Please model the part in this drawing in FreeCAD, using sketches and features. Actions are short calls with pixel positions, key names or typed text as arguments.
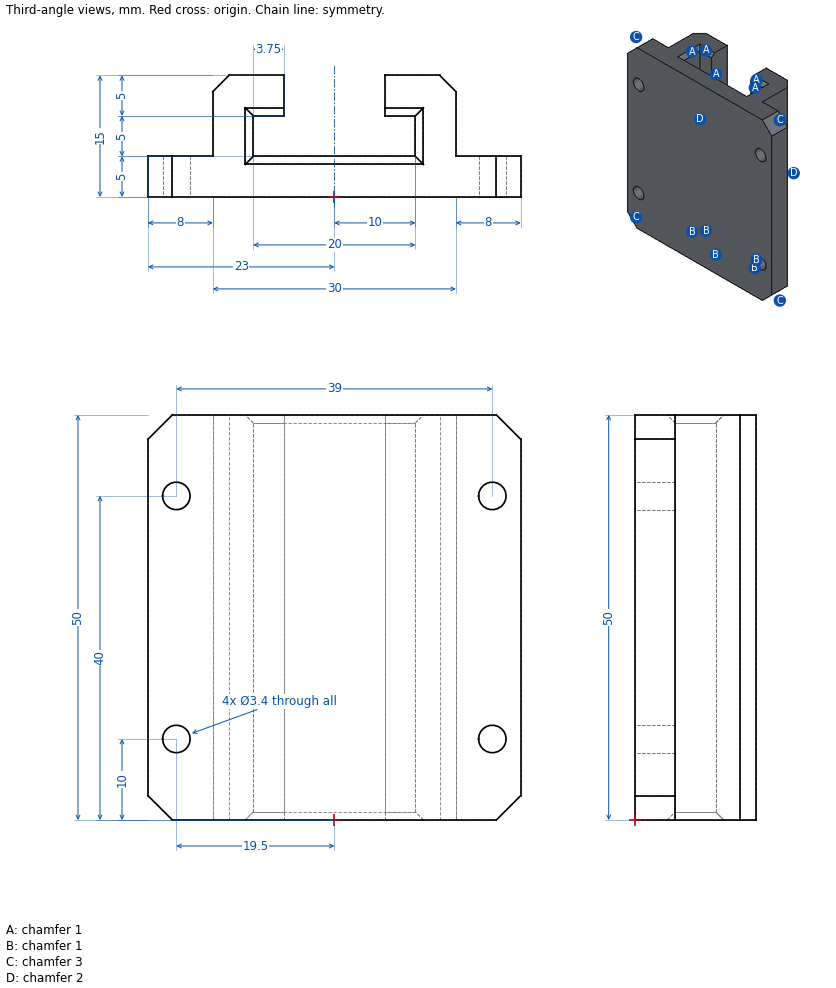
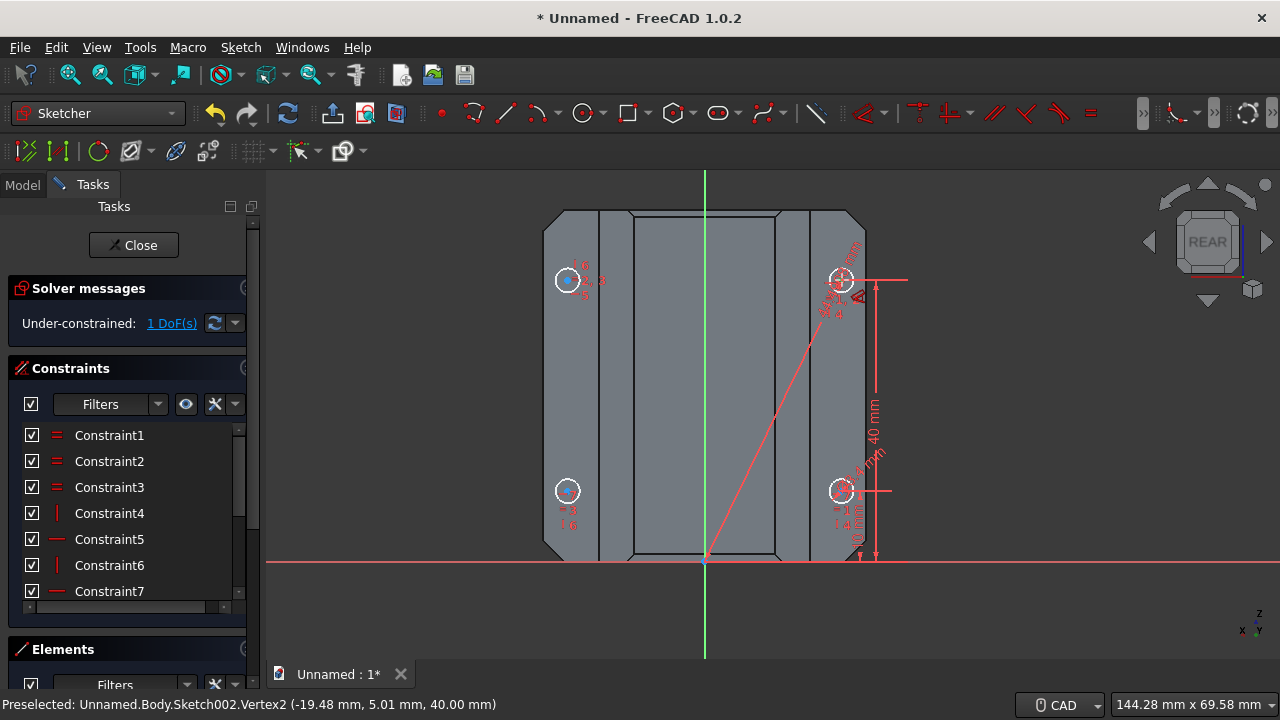
click(568, 280)
click(642, 246)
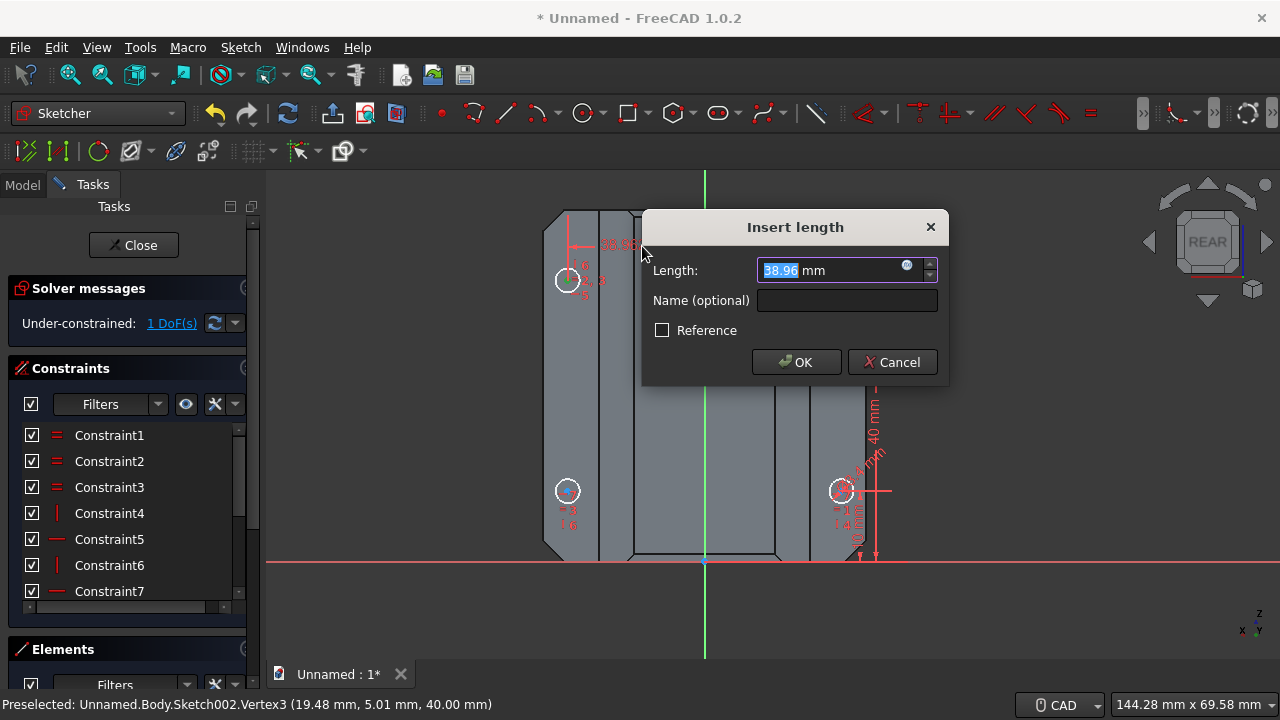
text(39)
key(Return)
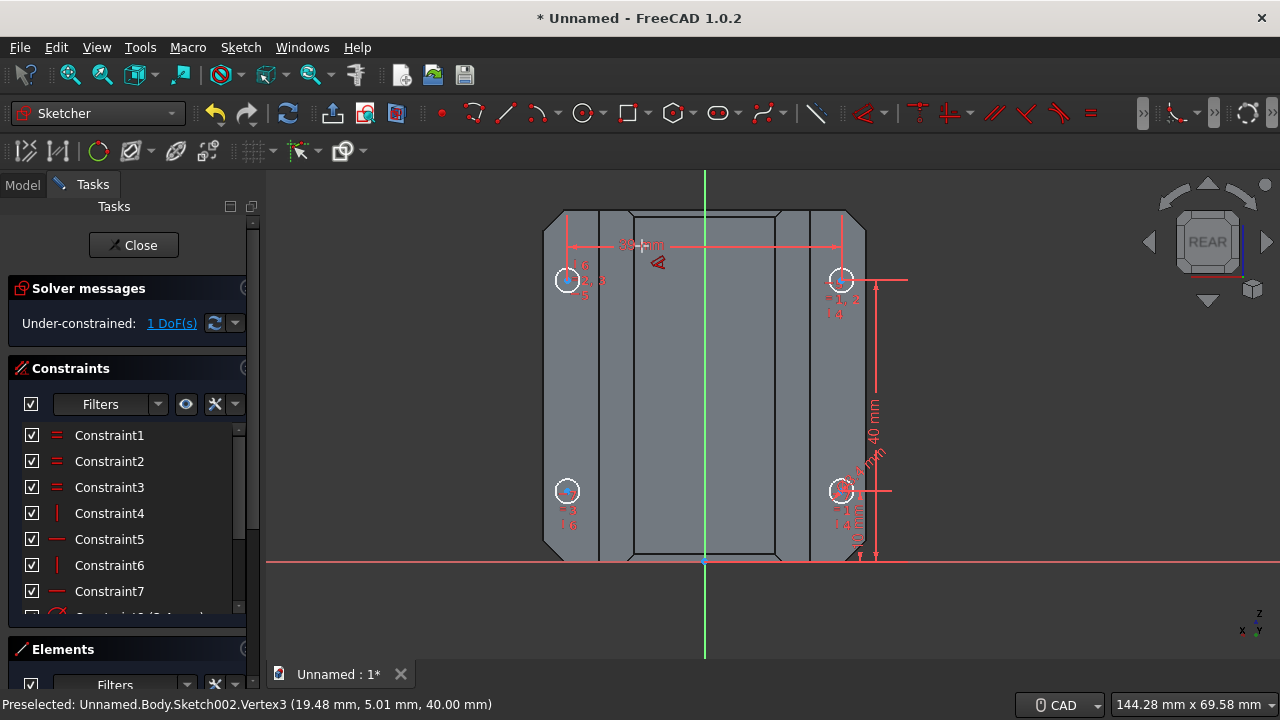
click(842, 491)
click(773, 596)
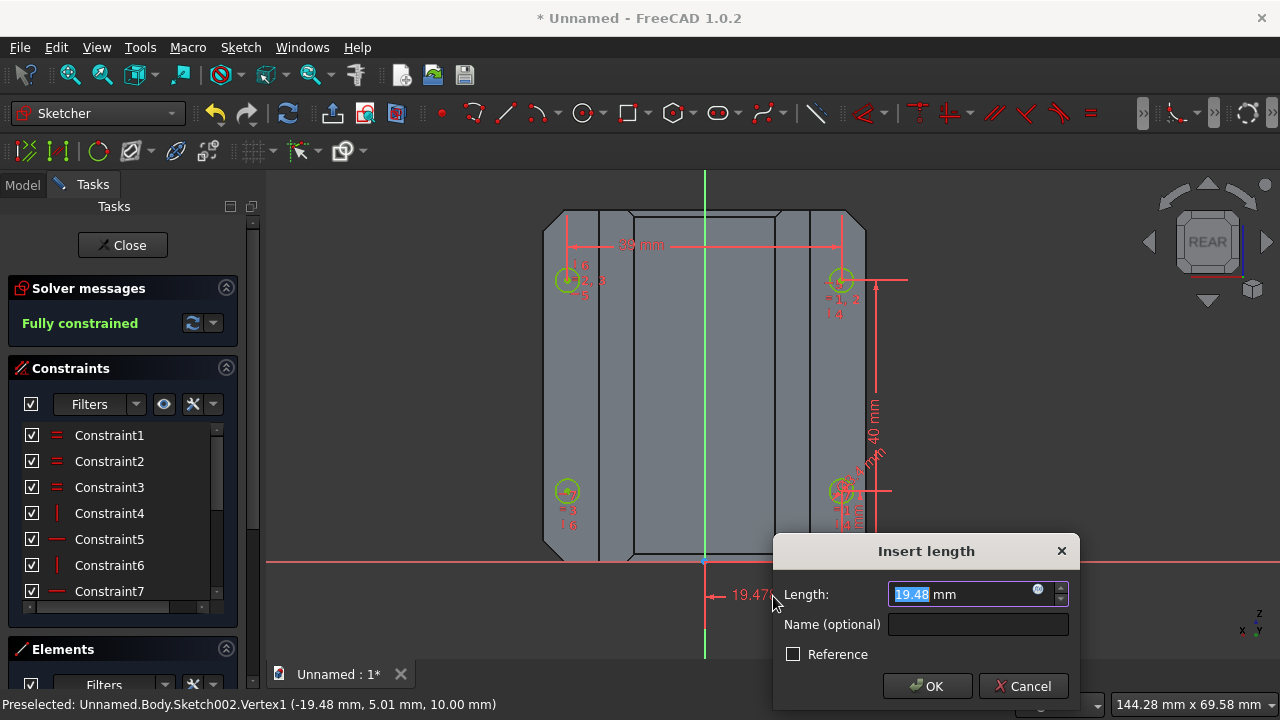
text(19.5)
key(Return)
key(Escape)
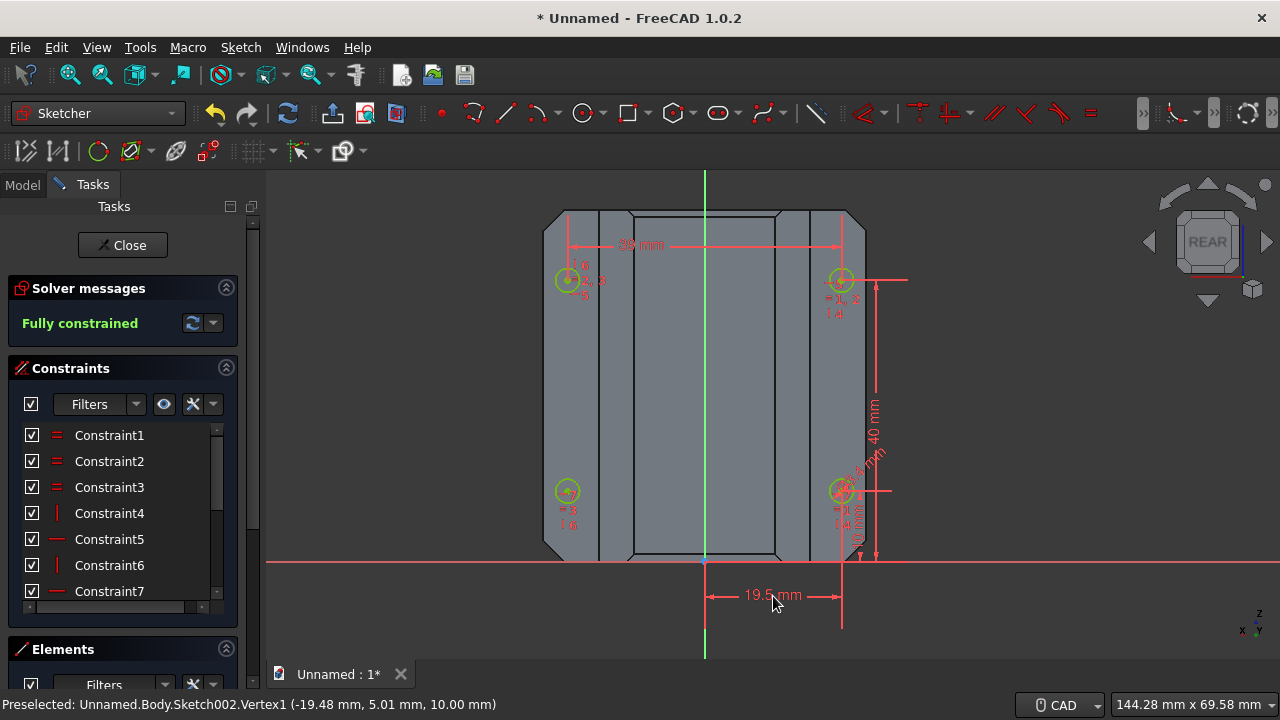
click(123, 245)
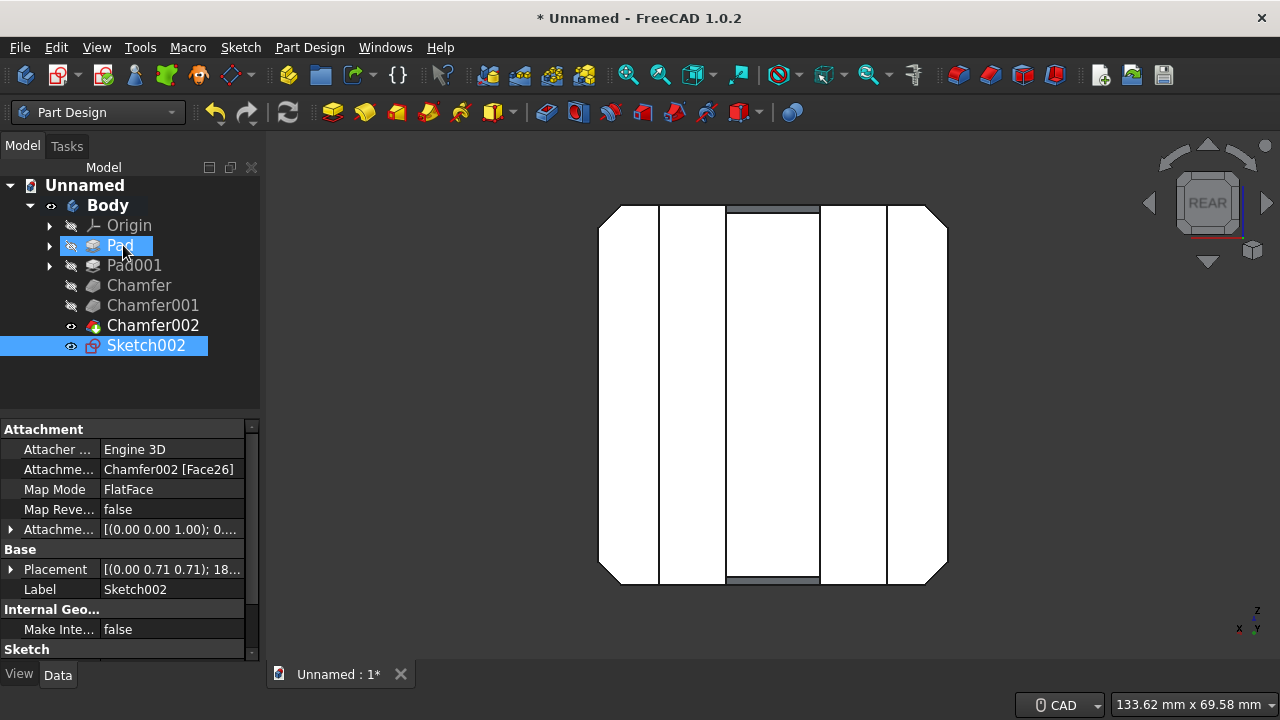
click(580, 112)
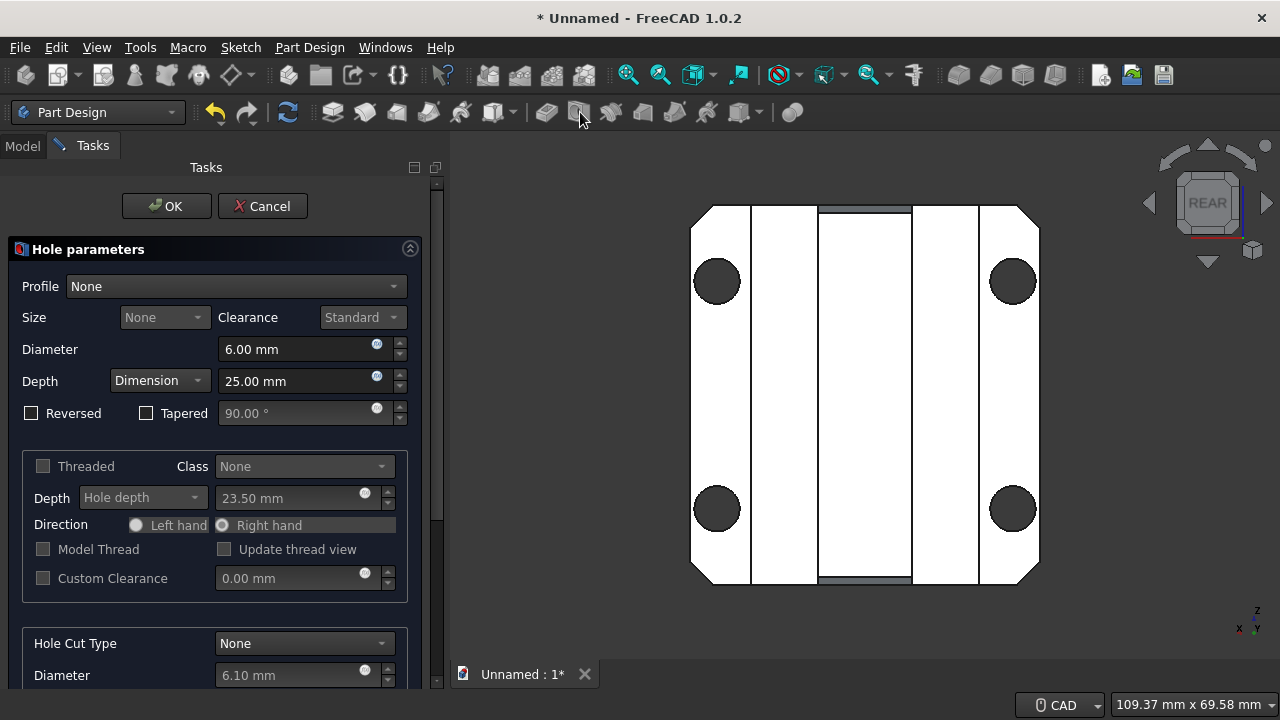
triple_click(305, 349)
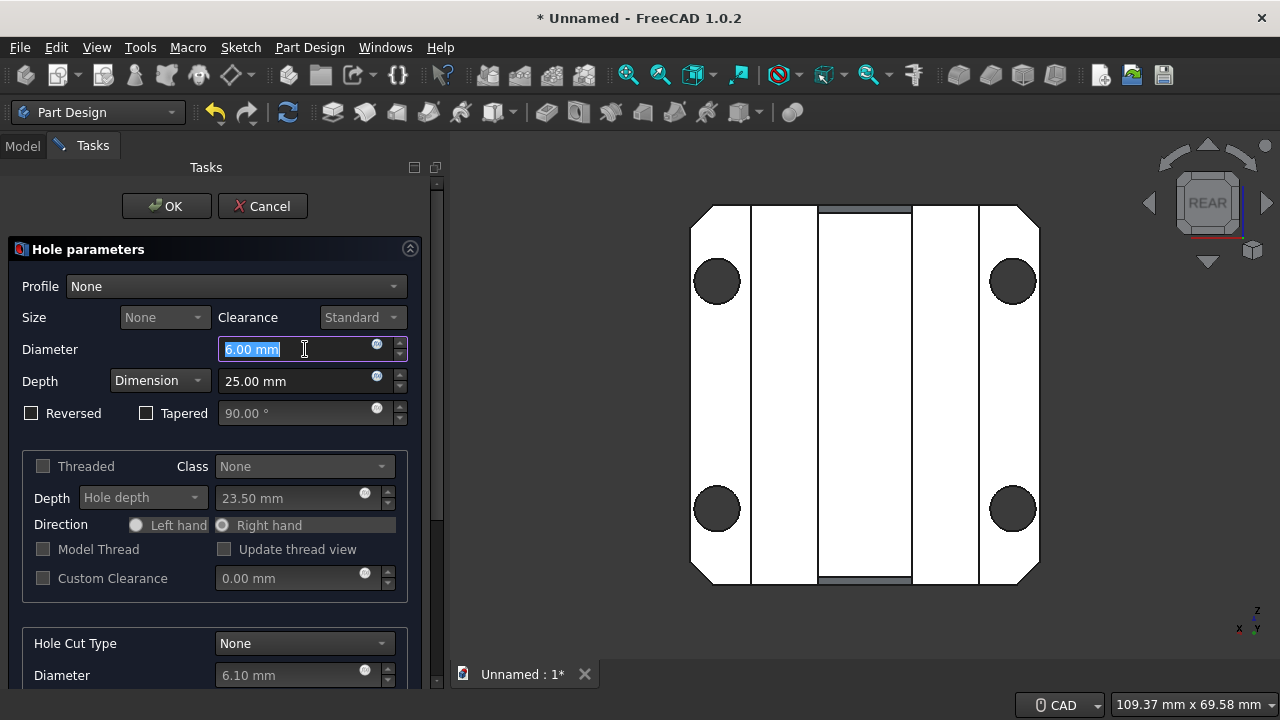
text(3.4)
key(Tab)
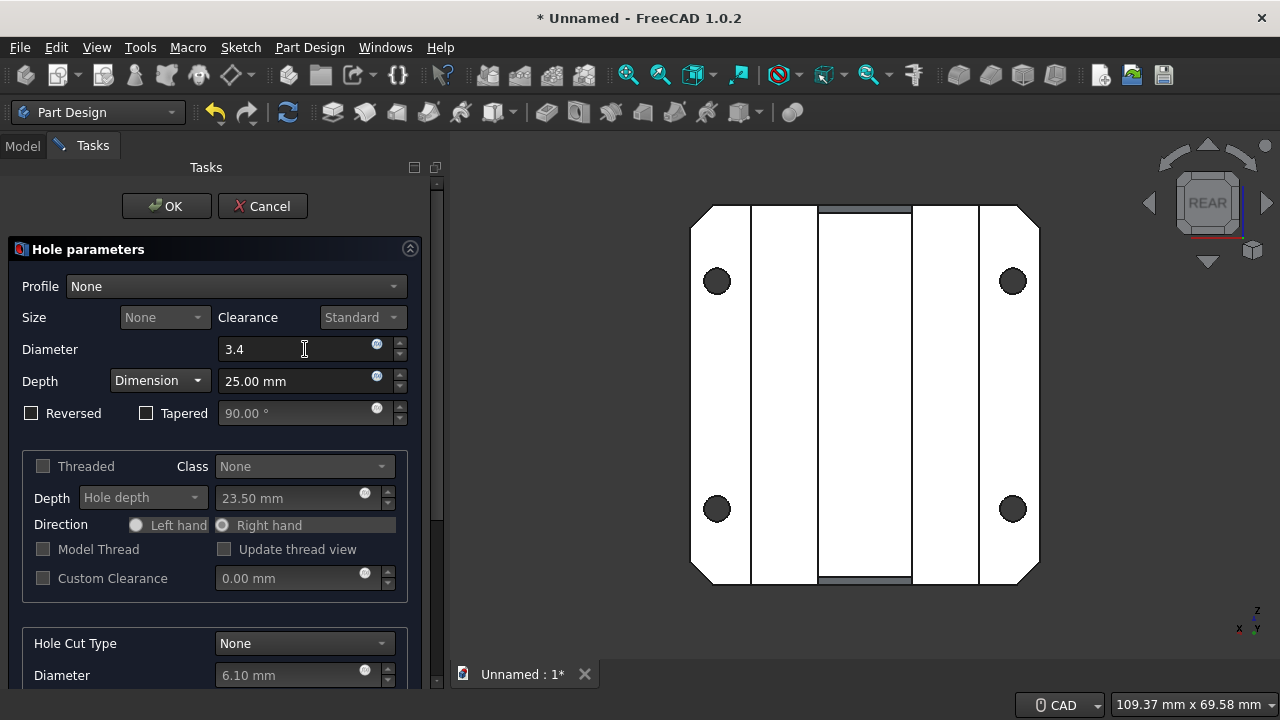
click(161, 380)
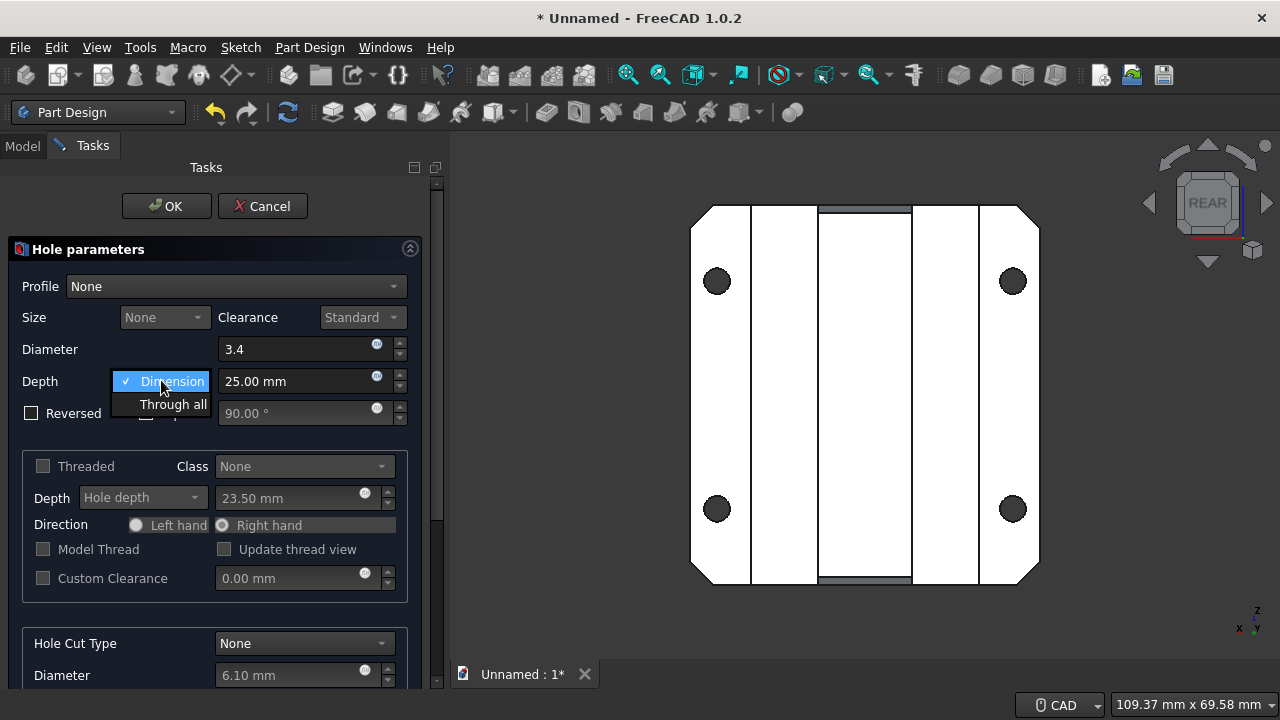
click(160, 404)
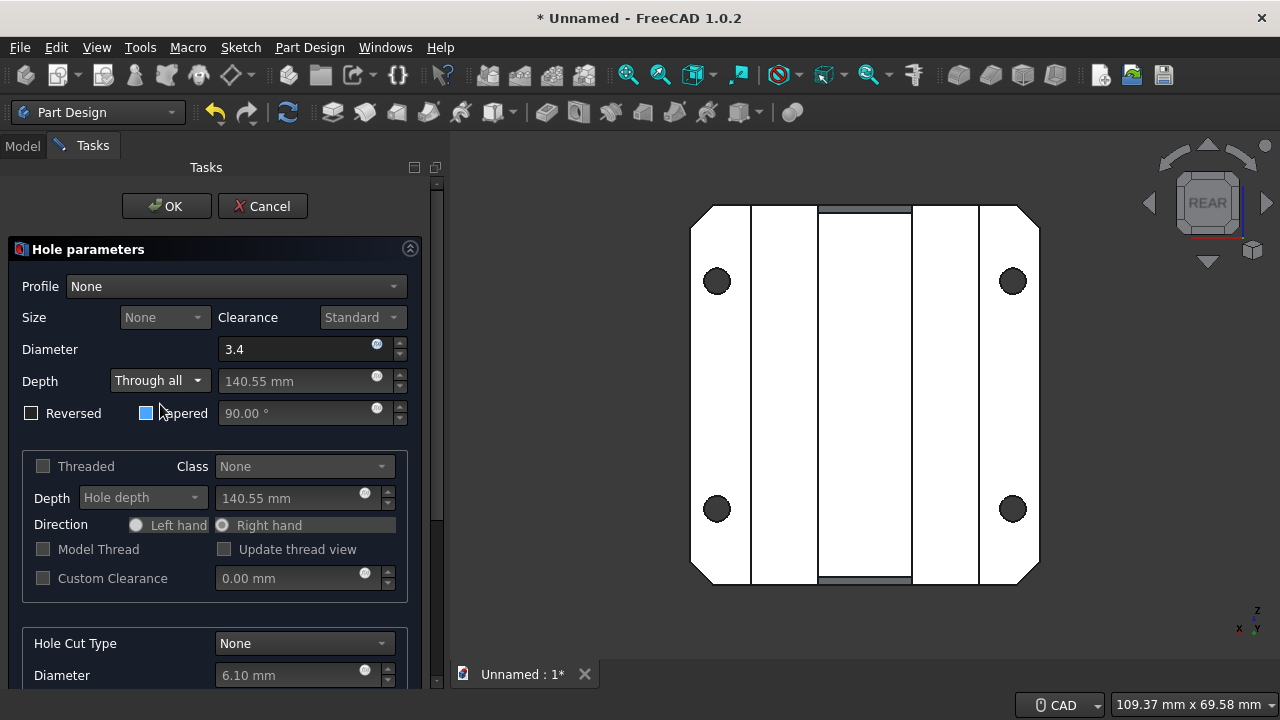
click(167, 206)